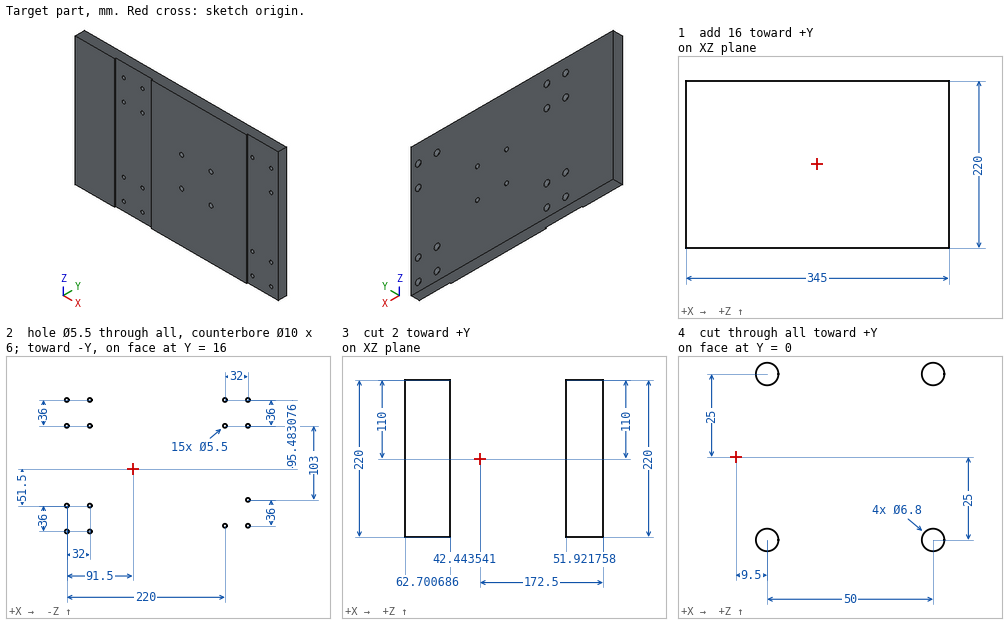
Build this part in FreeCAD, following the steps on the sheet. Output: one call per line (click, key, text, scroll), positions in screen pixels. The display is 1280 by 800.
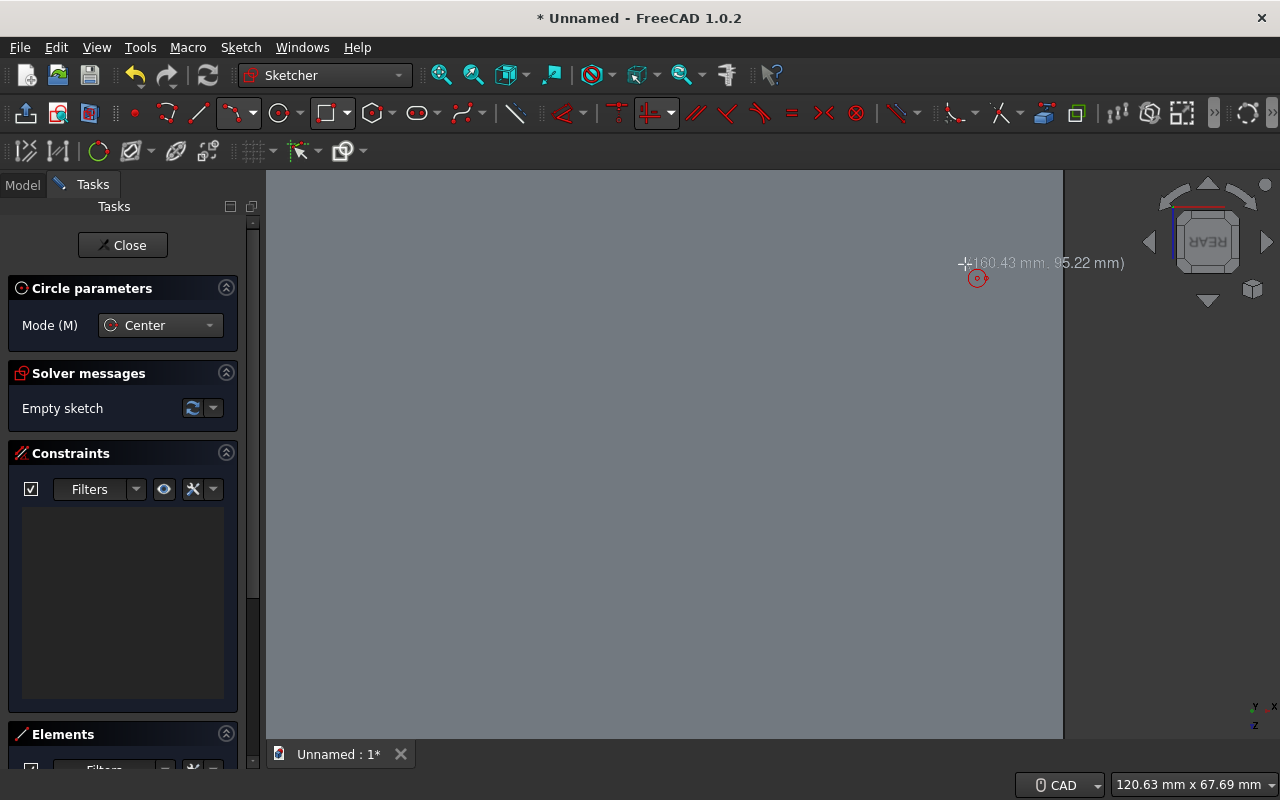
scroll(966, 265, down, 7)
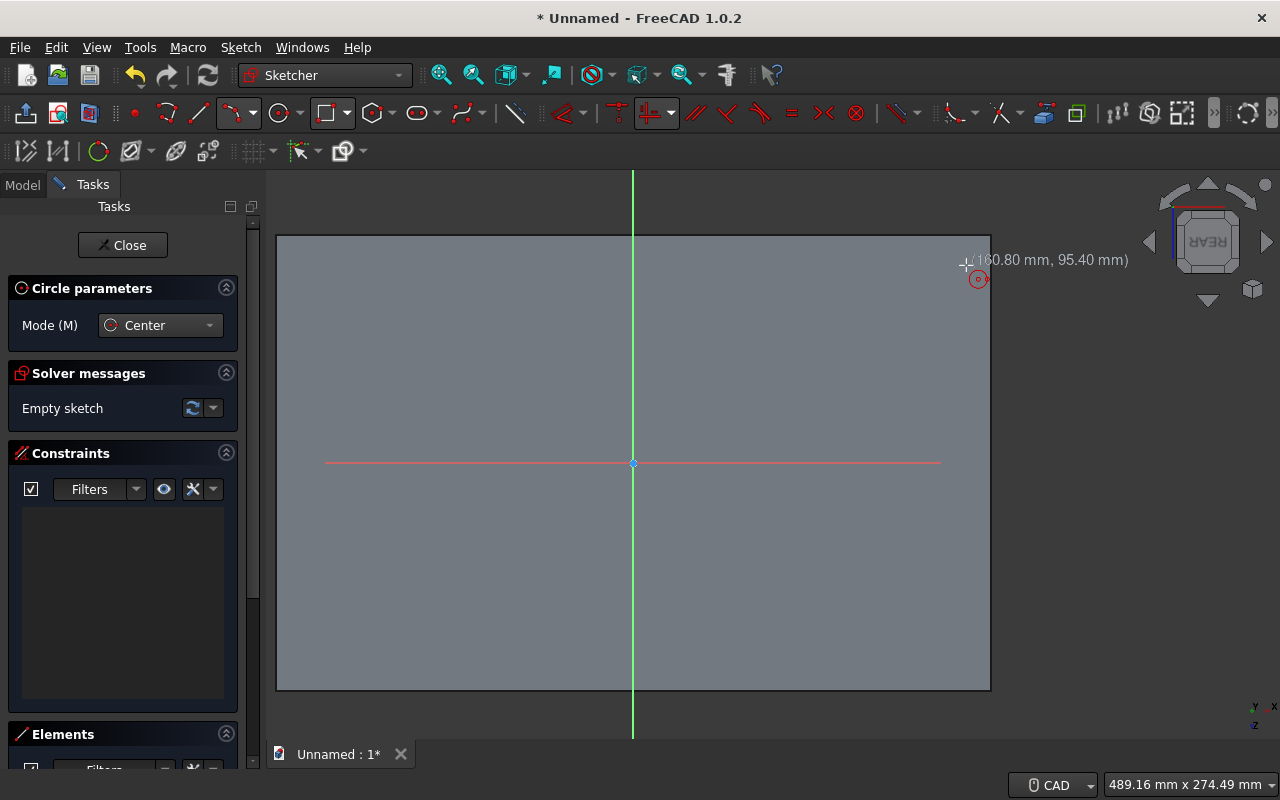
click(966, 265)
move(970, 261)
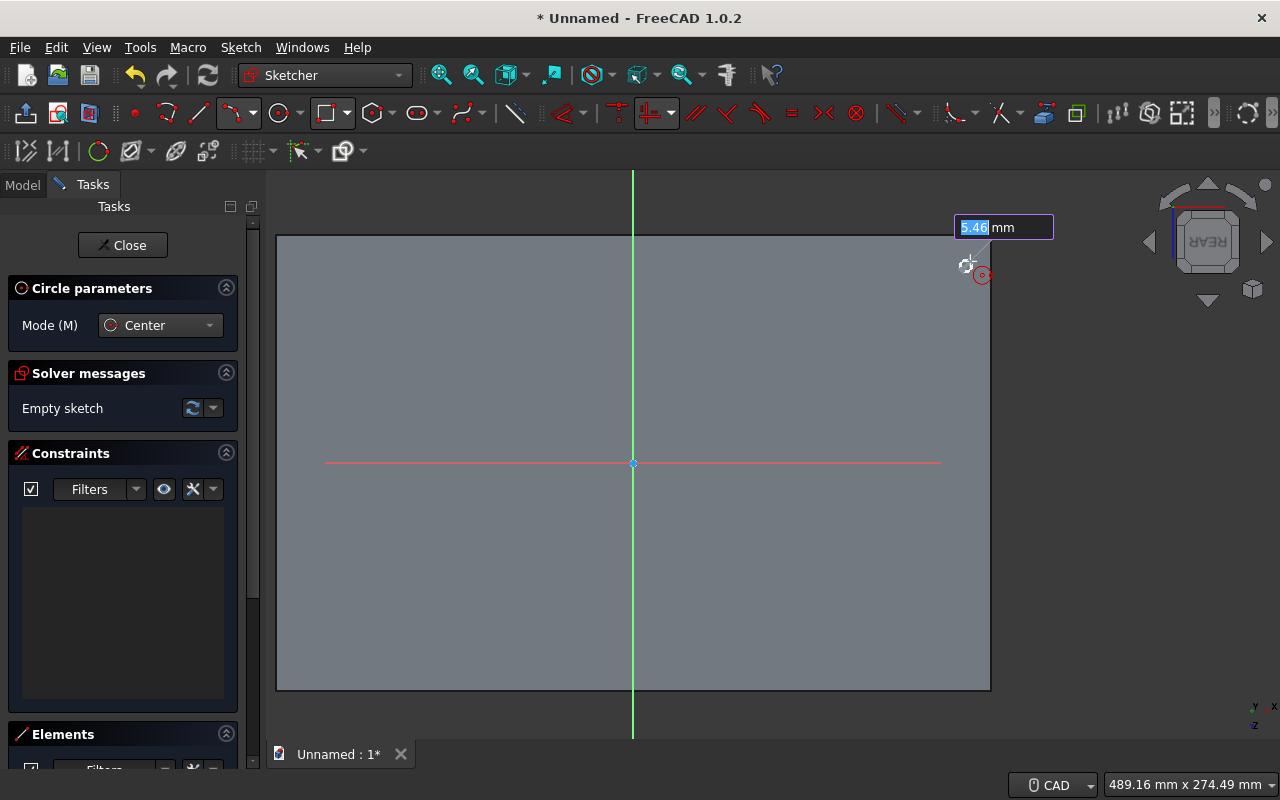
text(5.5)
key(Return)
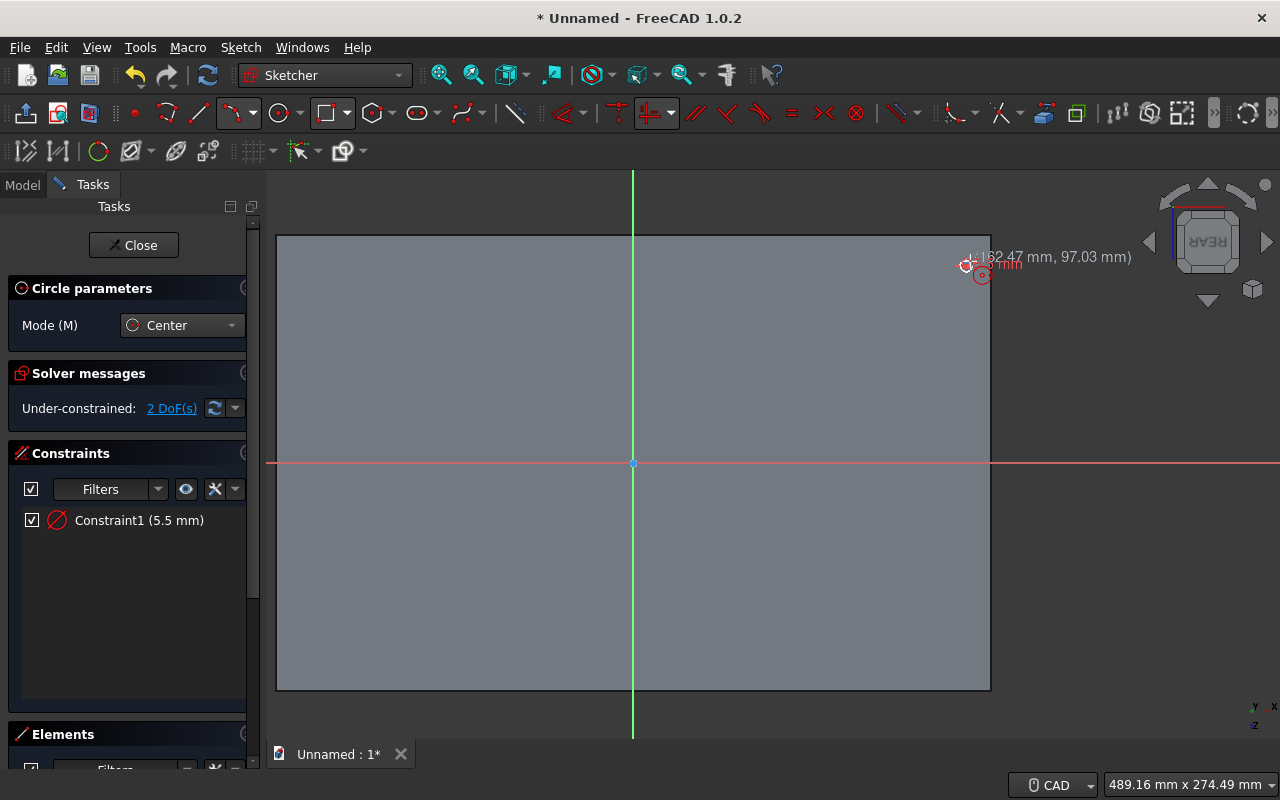
scroll(900, 265, up, 7)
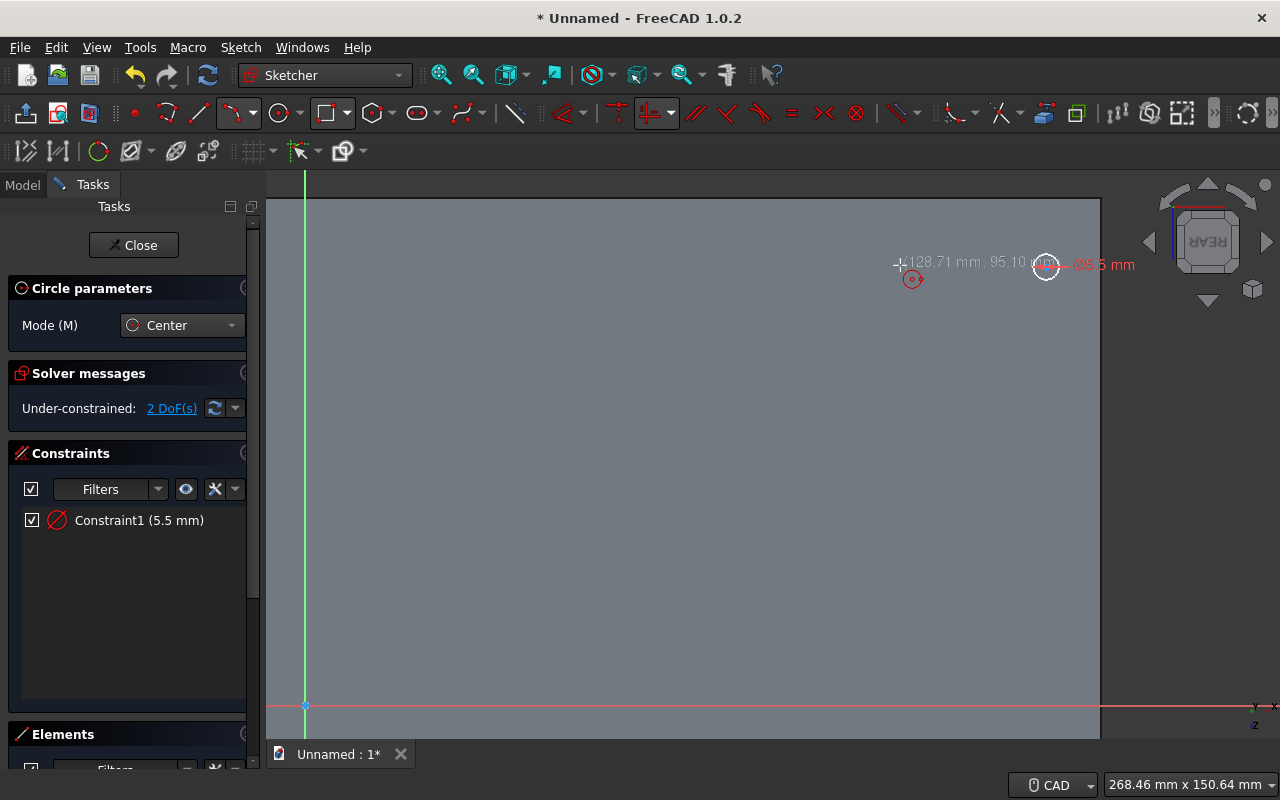
scroll(900, 265, down, 7)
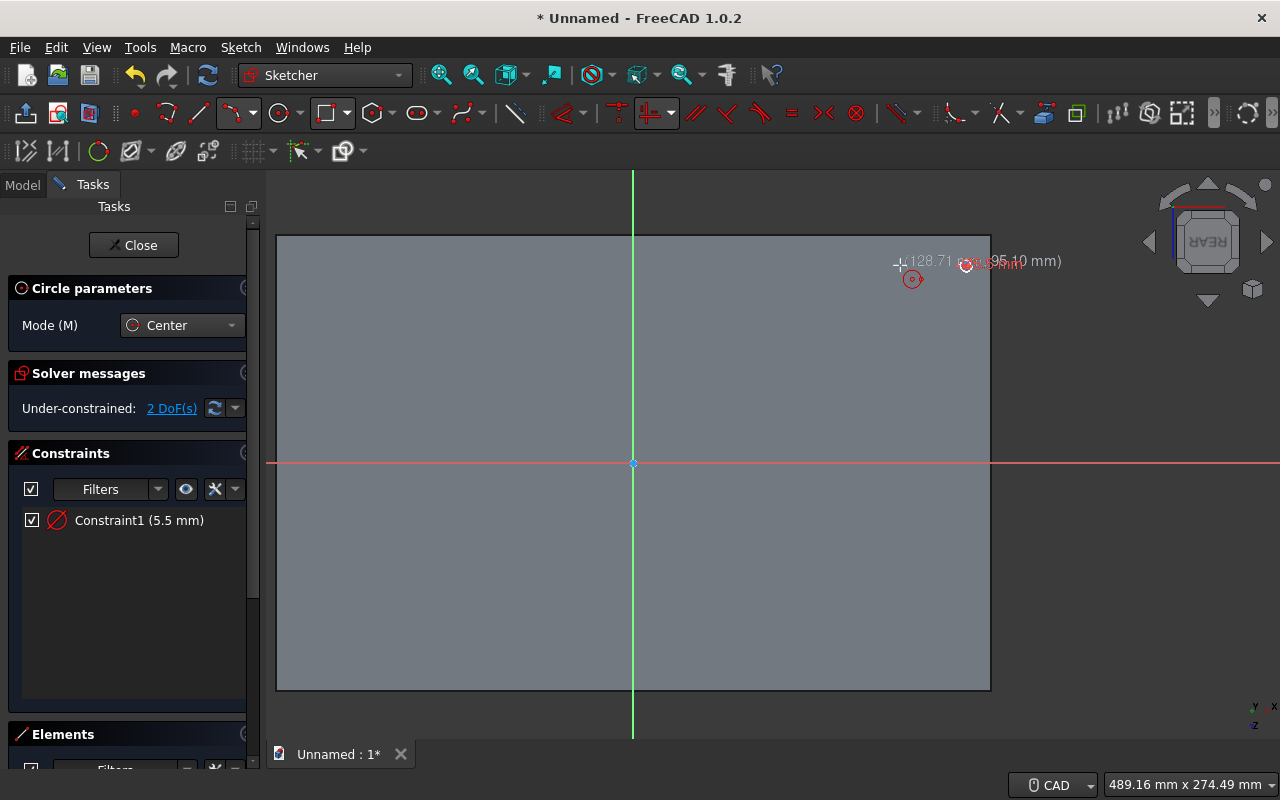
click(900, 265)
move(904, 261)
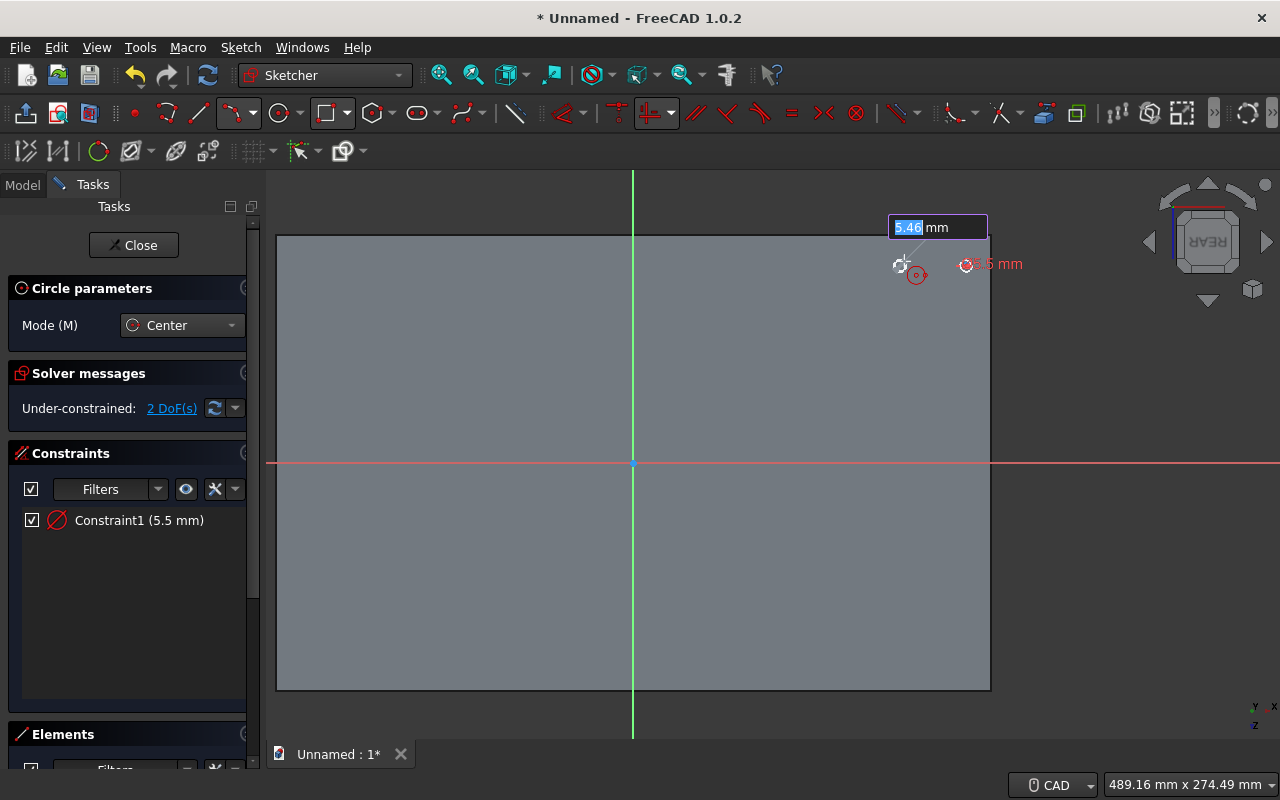
text(5.5)
key(Return)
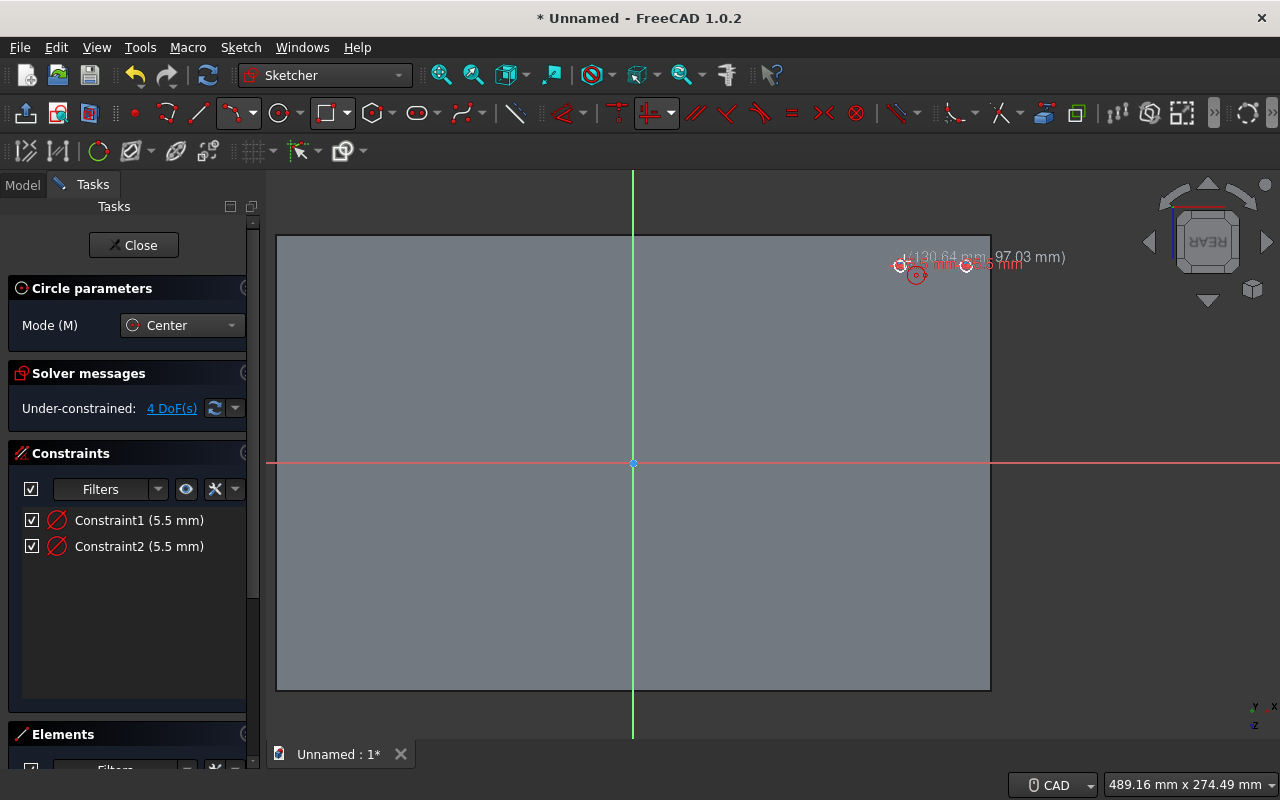
scroll(900, 340, up, 7)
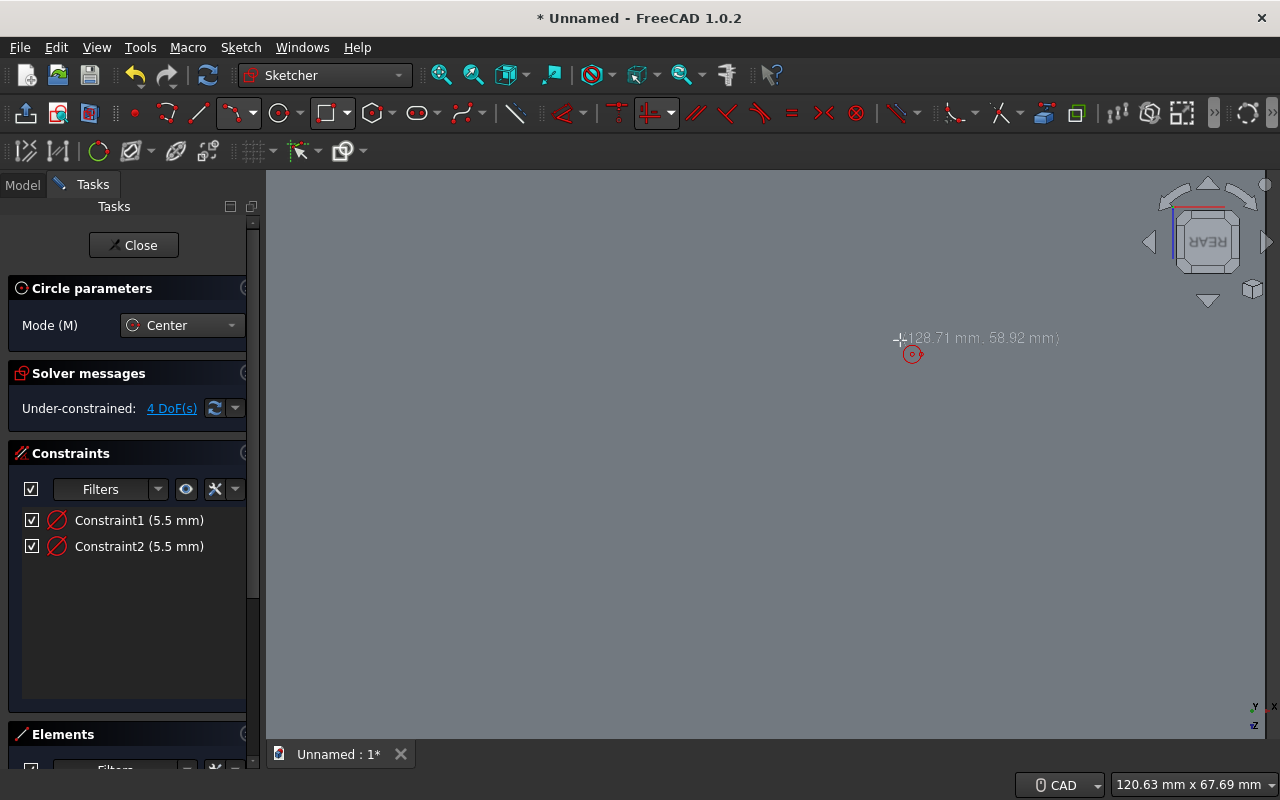
scroll(900, 340, down, 7)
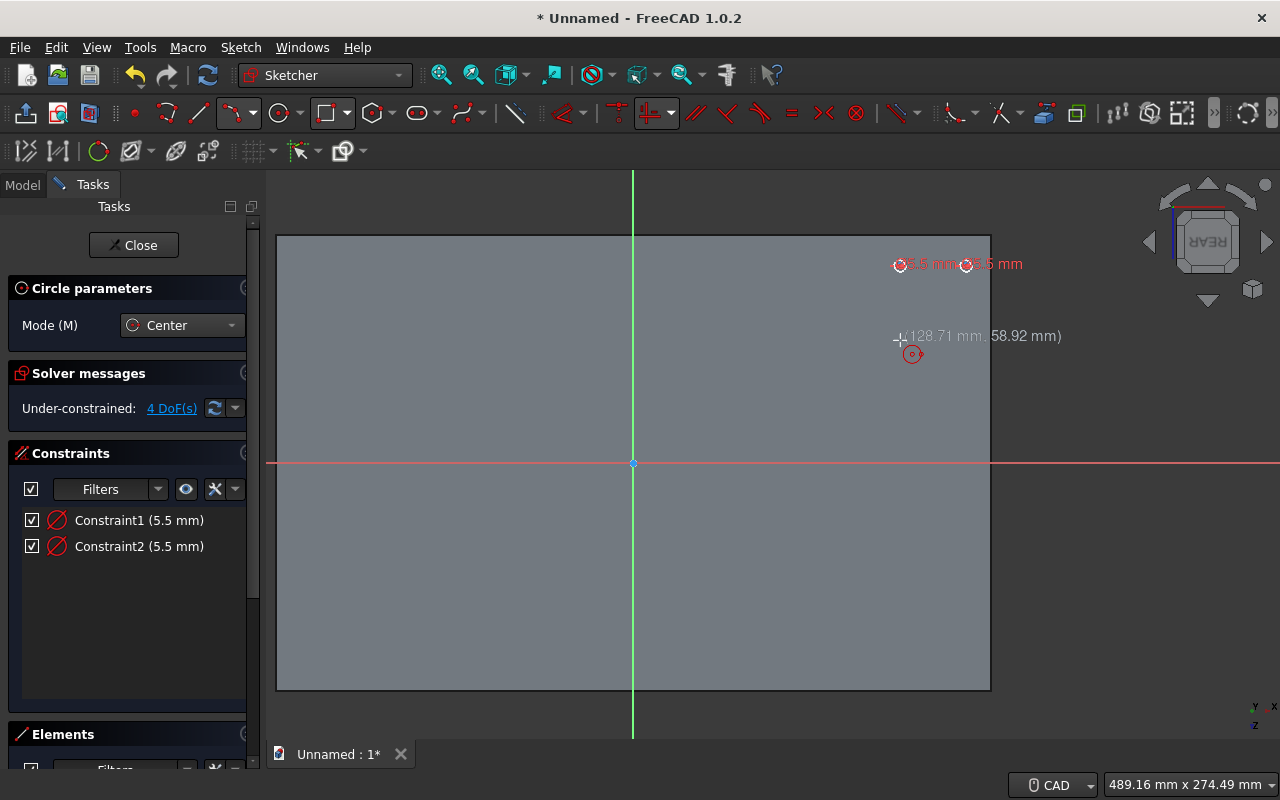
click(900, 340)
move(904, 336)